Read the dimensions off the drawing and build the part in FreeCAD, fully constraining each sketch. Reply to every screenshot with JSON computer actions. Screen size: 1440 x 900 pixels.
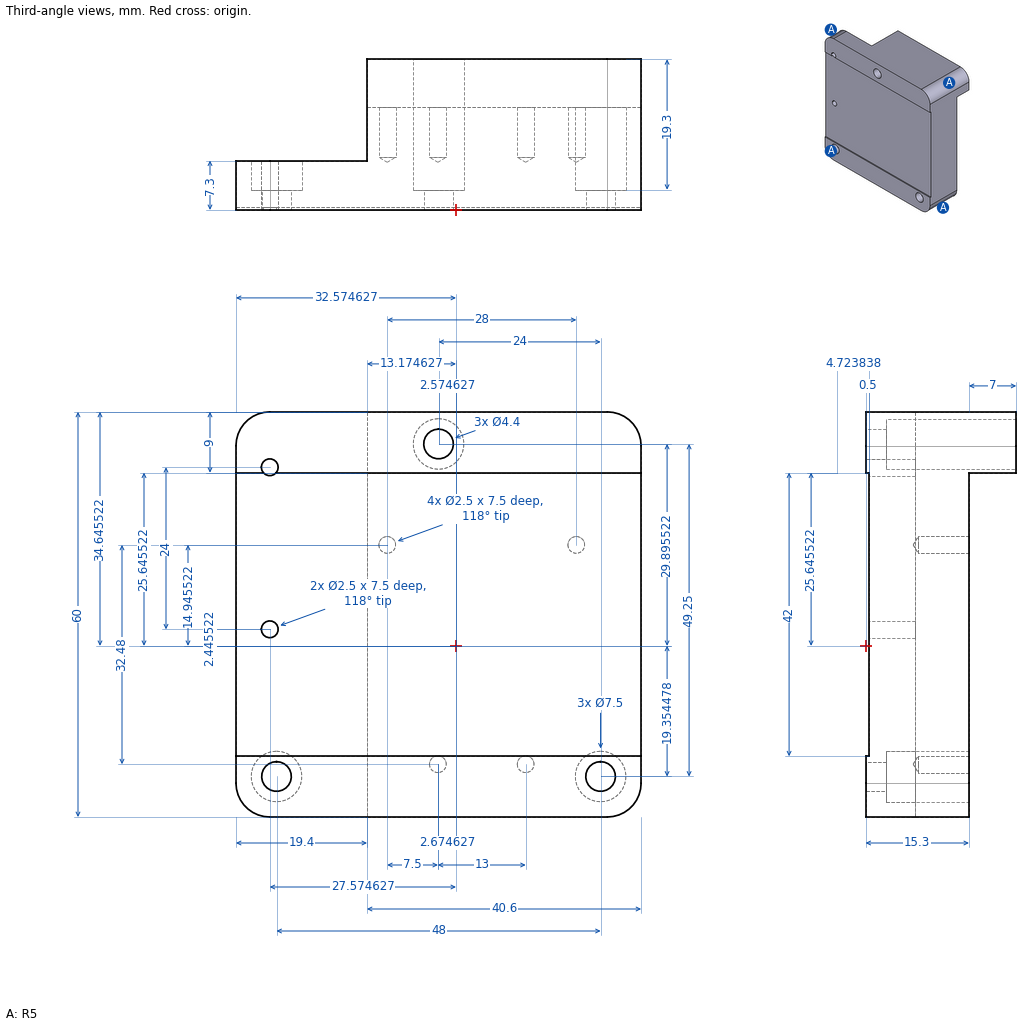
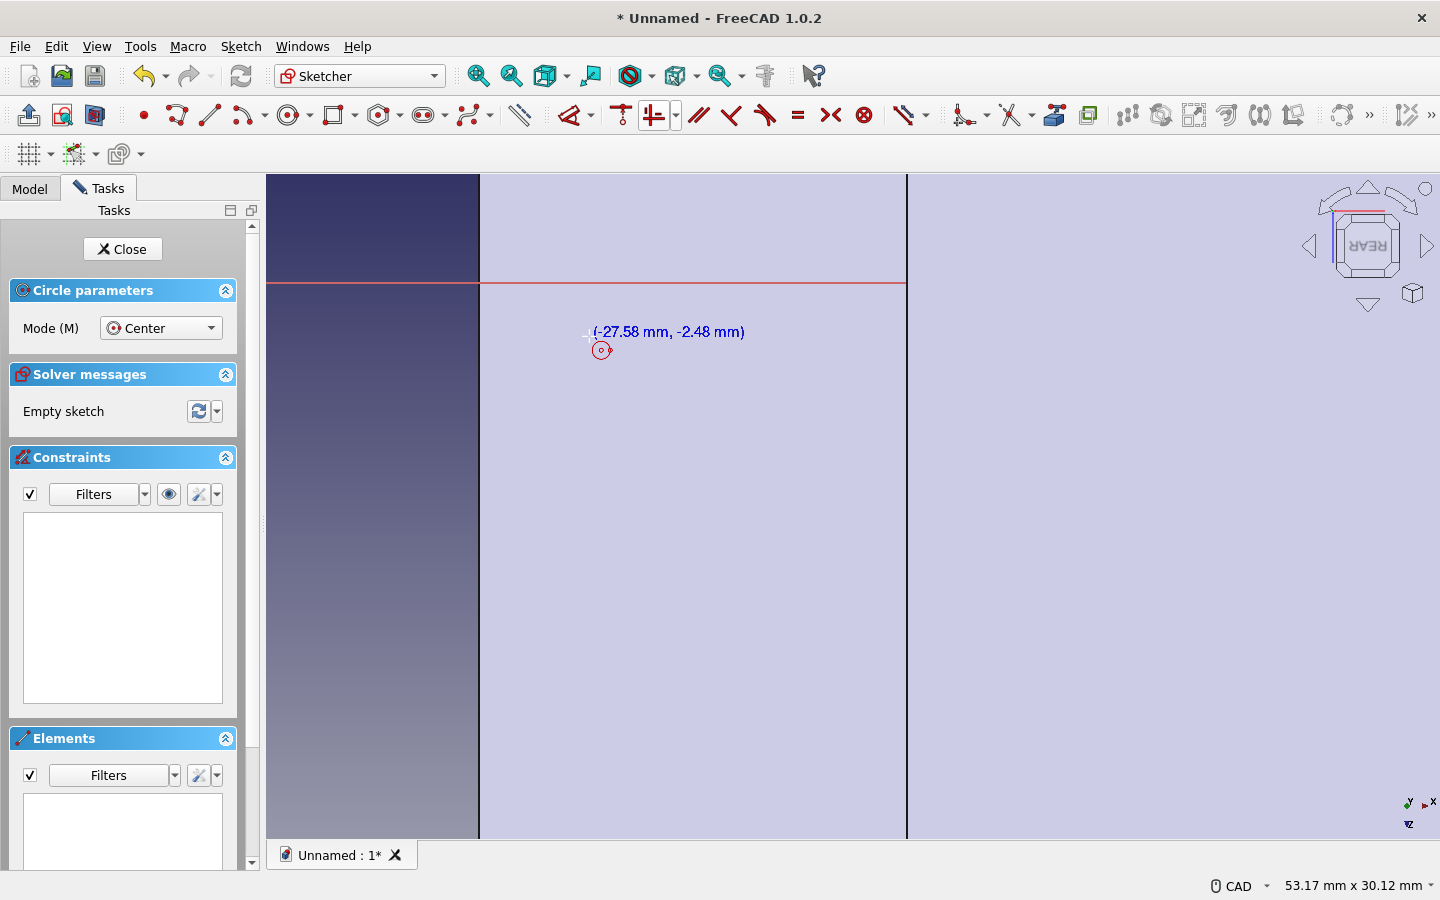
{"action": "left_click", "coordinate": [589, 337]}
{"action": "left_click", "coordinate": [608, 317]}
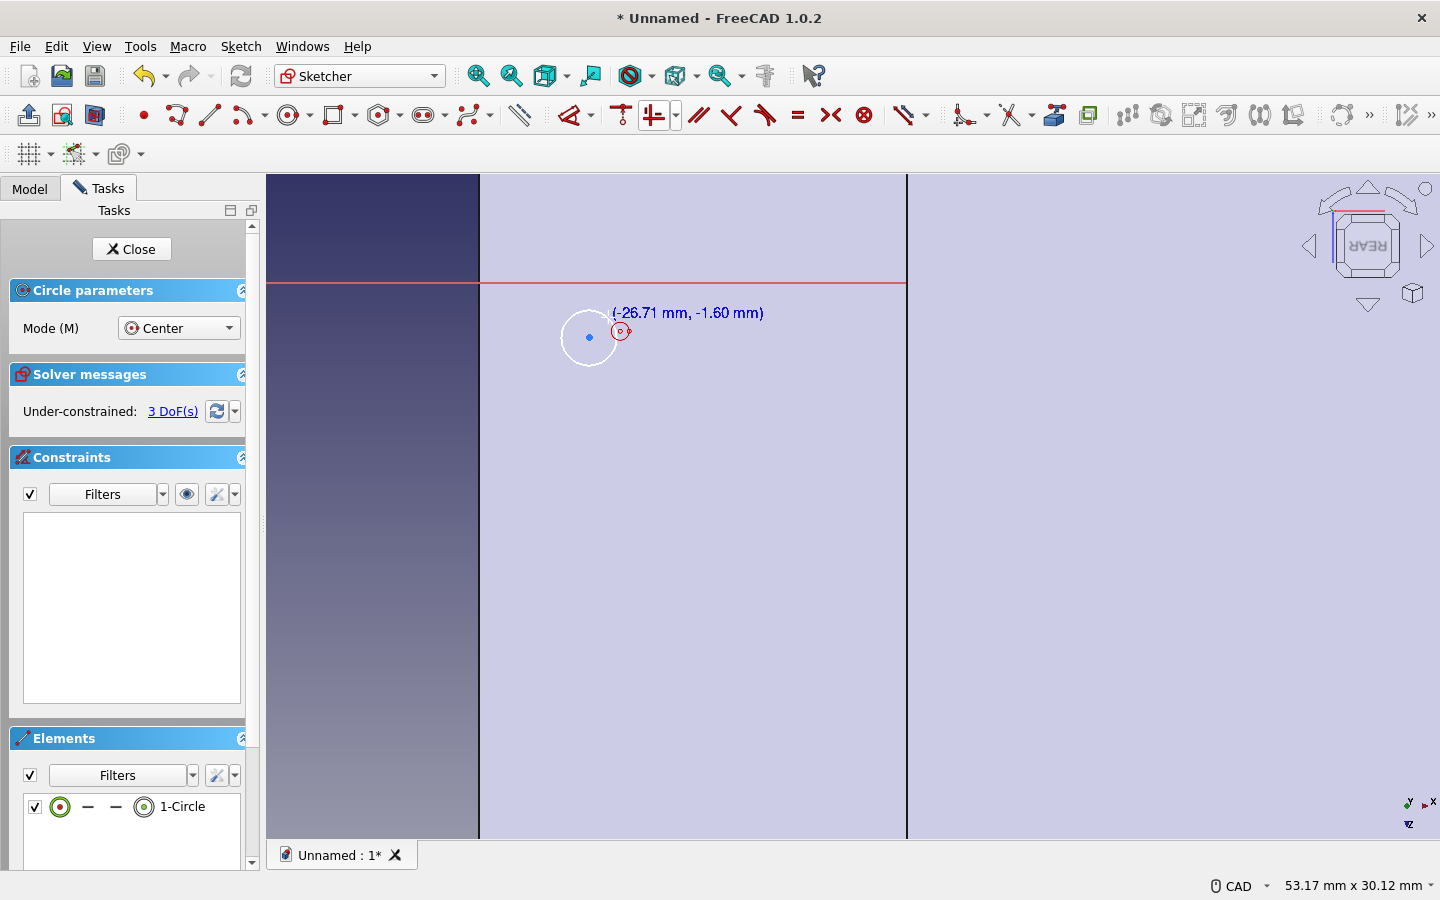
{"action": "scroll", "coordinate": [591, 340], "scroll_direction": "down", "scroll_amount": 2}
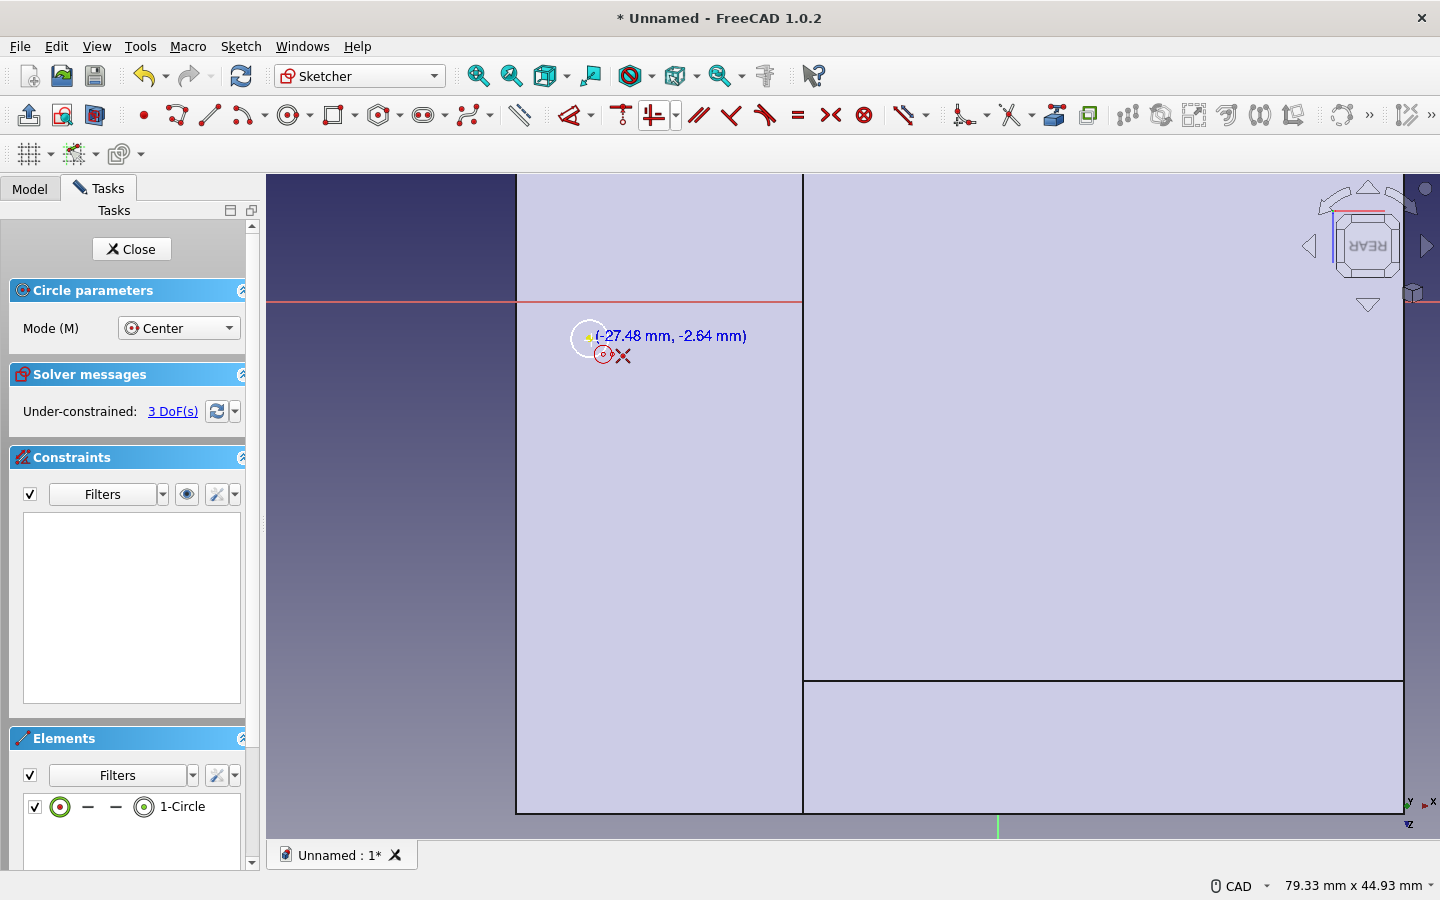
{"action": "scroll", "coordinate": [590, 693], "scroll_direction": "up", "scroll_amount": 2}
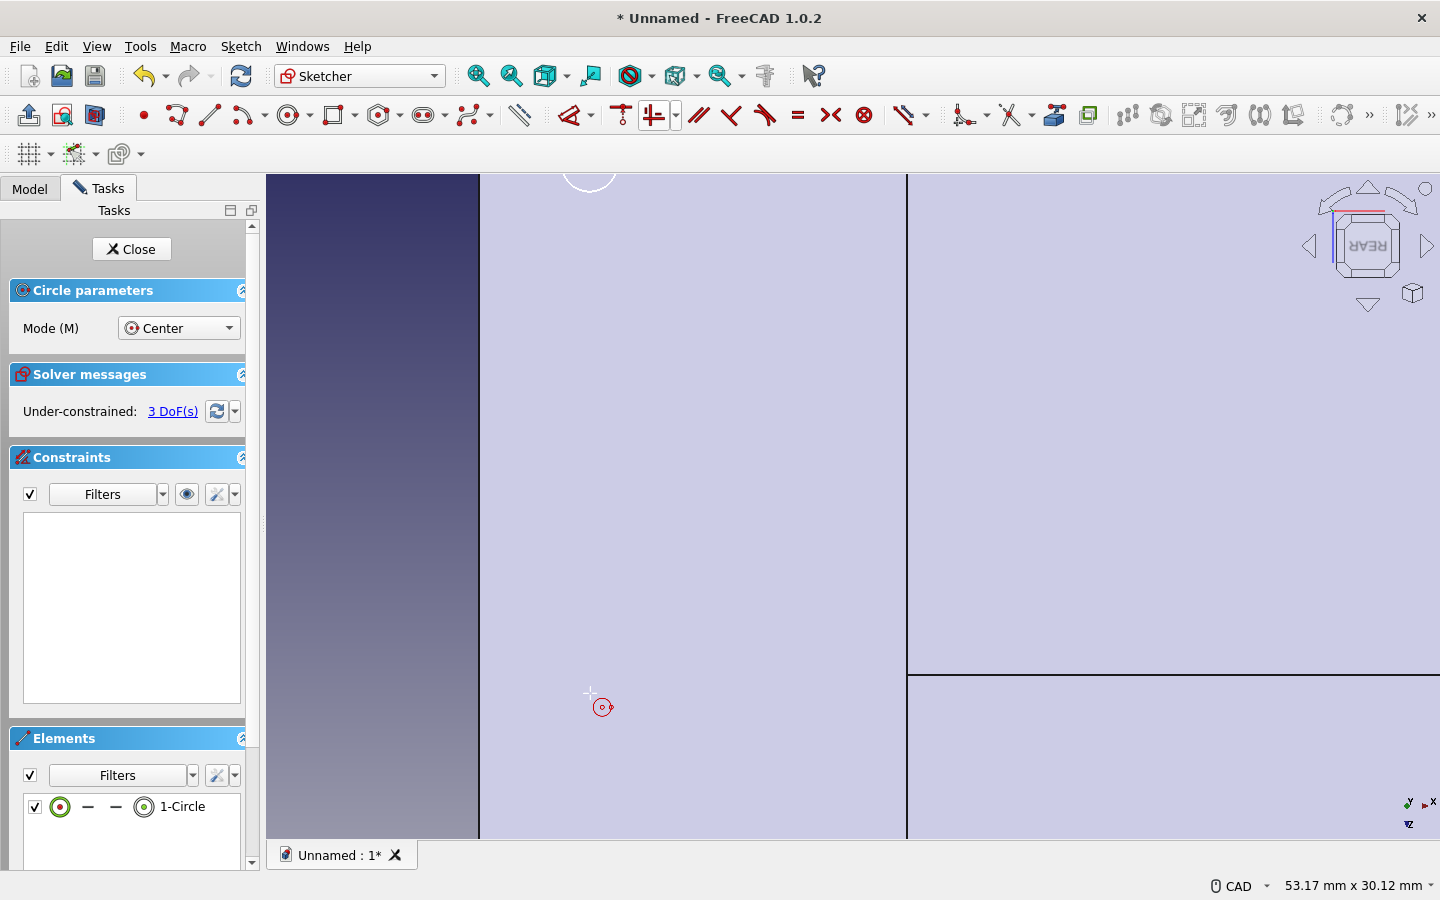
{"action": "left_click", "coordinate": [589, 693]}
{"action": "left_click", "coordinate": [609, 673]}
{"action": "key", "text": "Escape"}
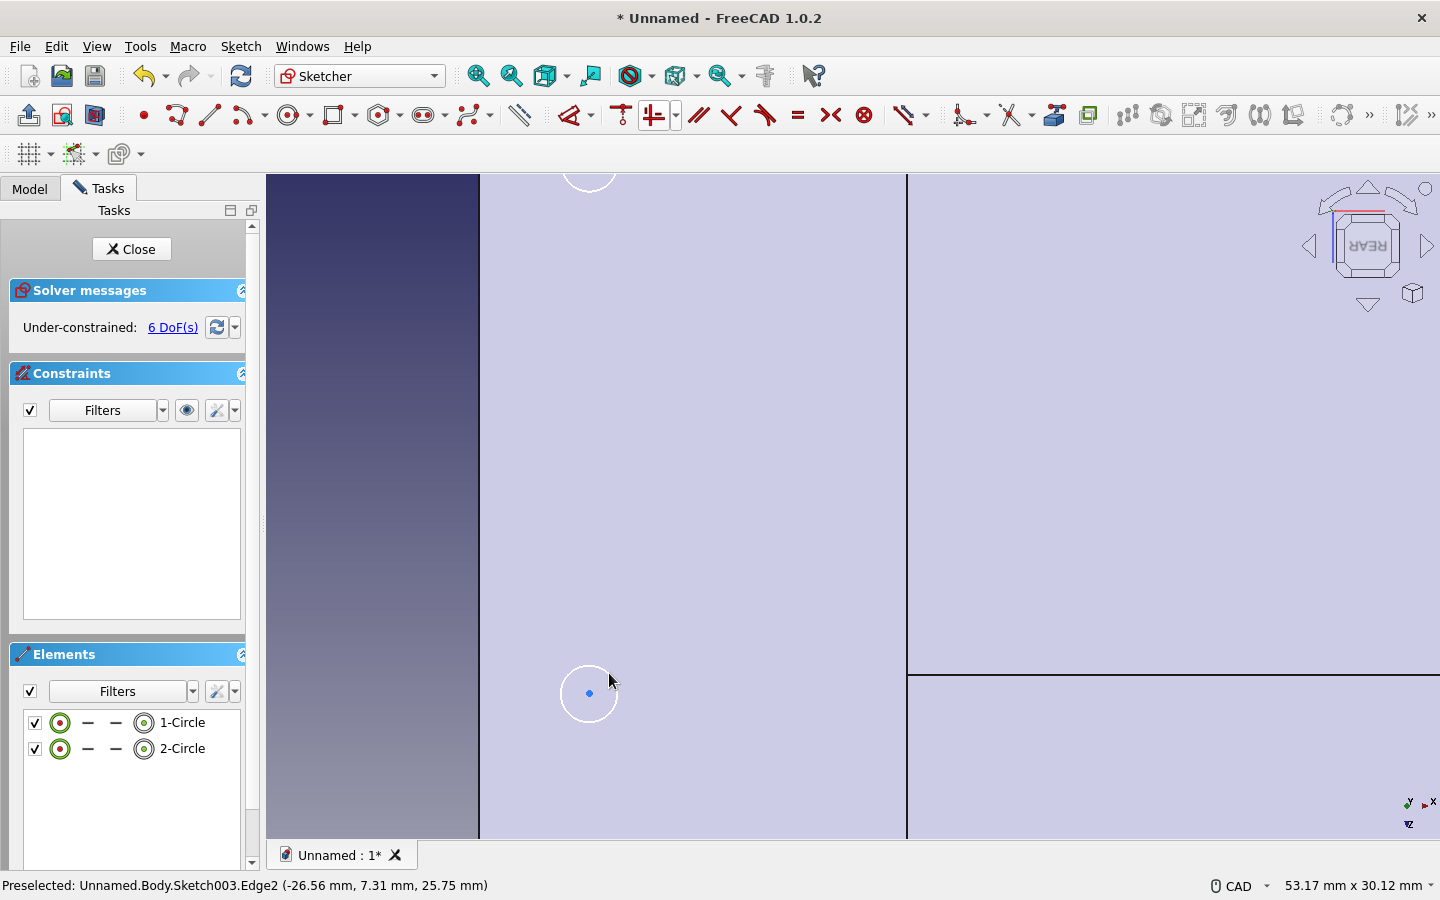
{"action": "scroll", "coordinate": [590, 694], "scroll_direction": "down", "scroll_amount": 2}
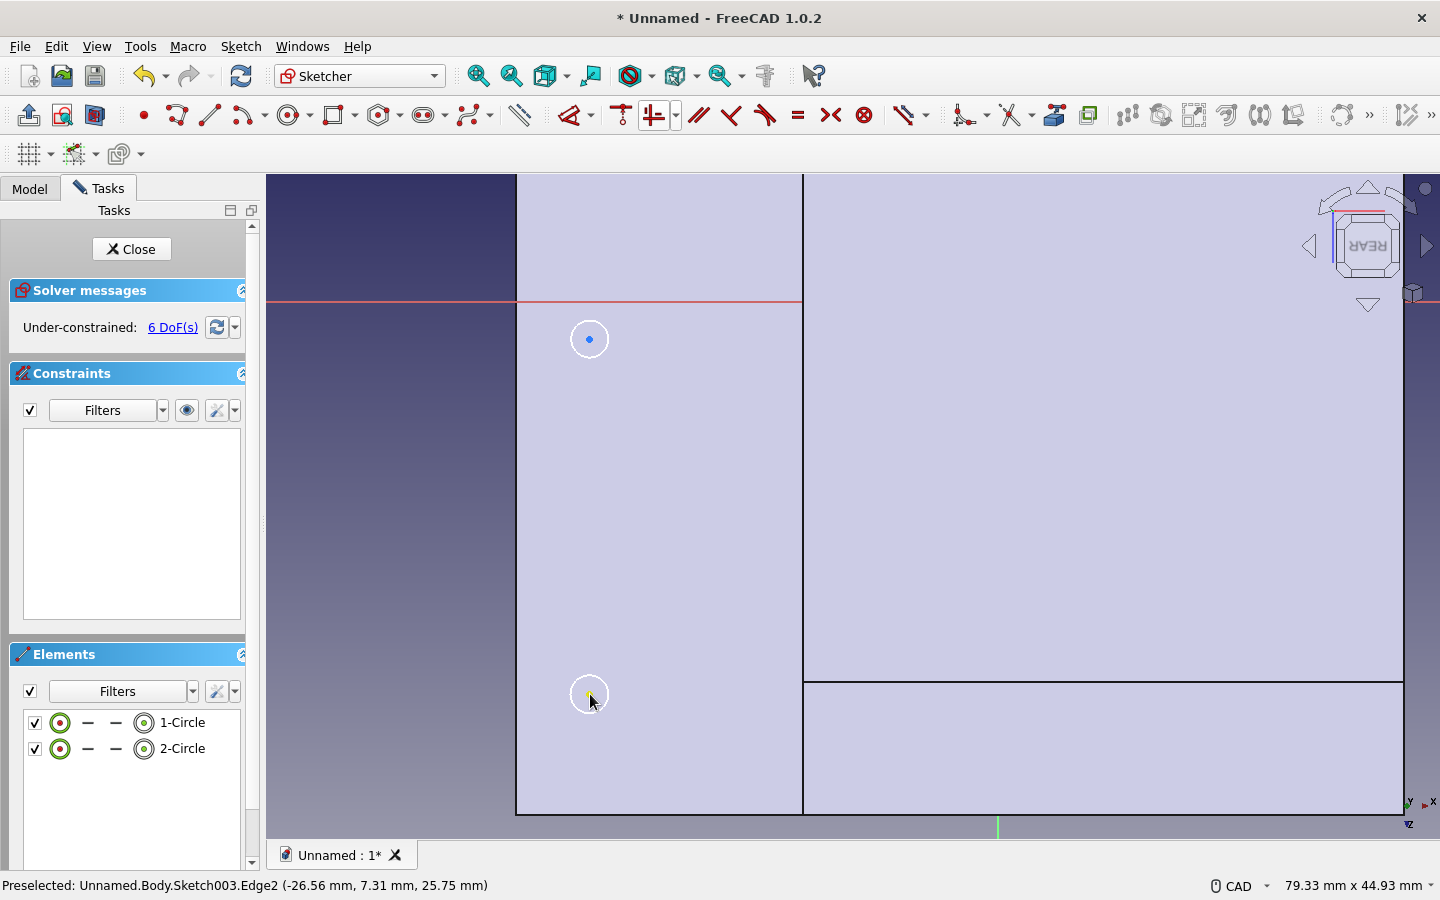
{"action": "left_click", "coordinate": [603, 326]}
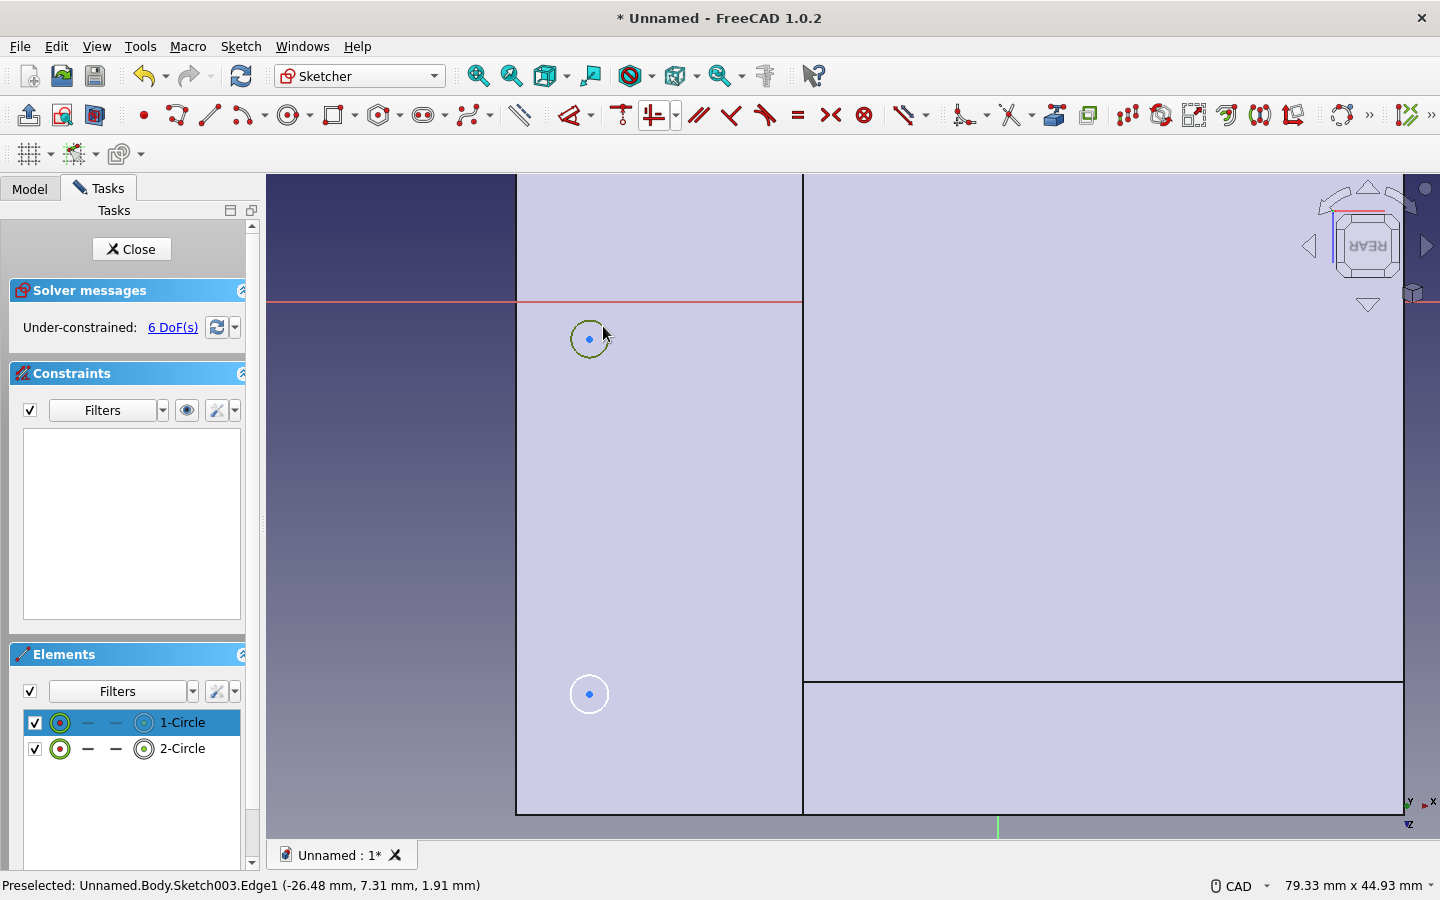
{"action": "left_click", "coordinate": [603, 681]}